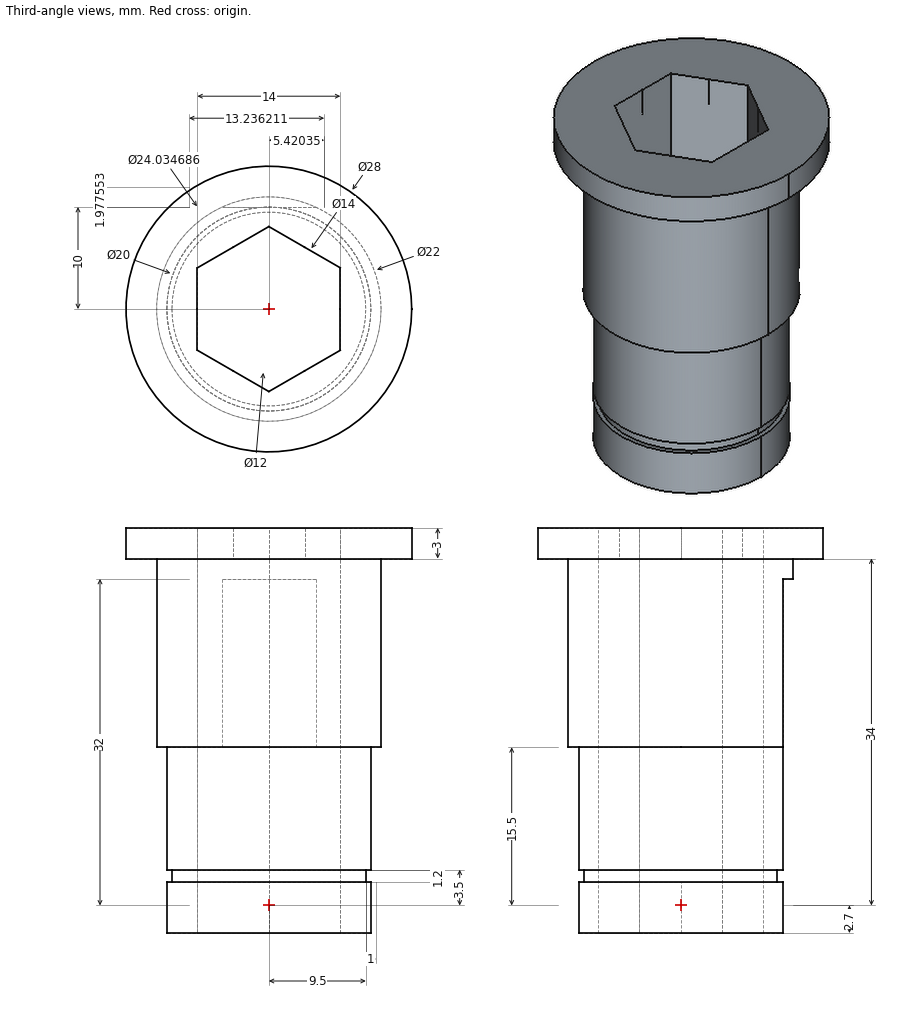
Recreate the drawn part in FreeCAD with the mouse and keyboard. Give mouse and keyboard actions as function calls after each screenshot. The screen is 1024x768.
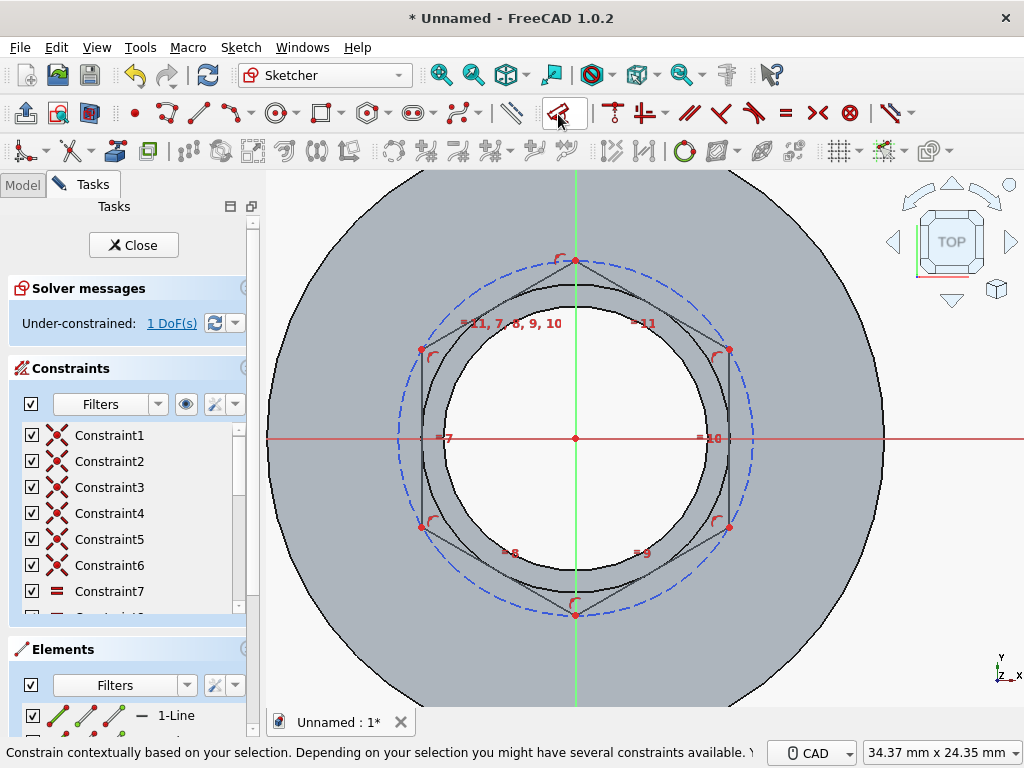
click(422, 350)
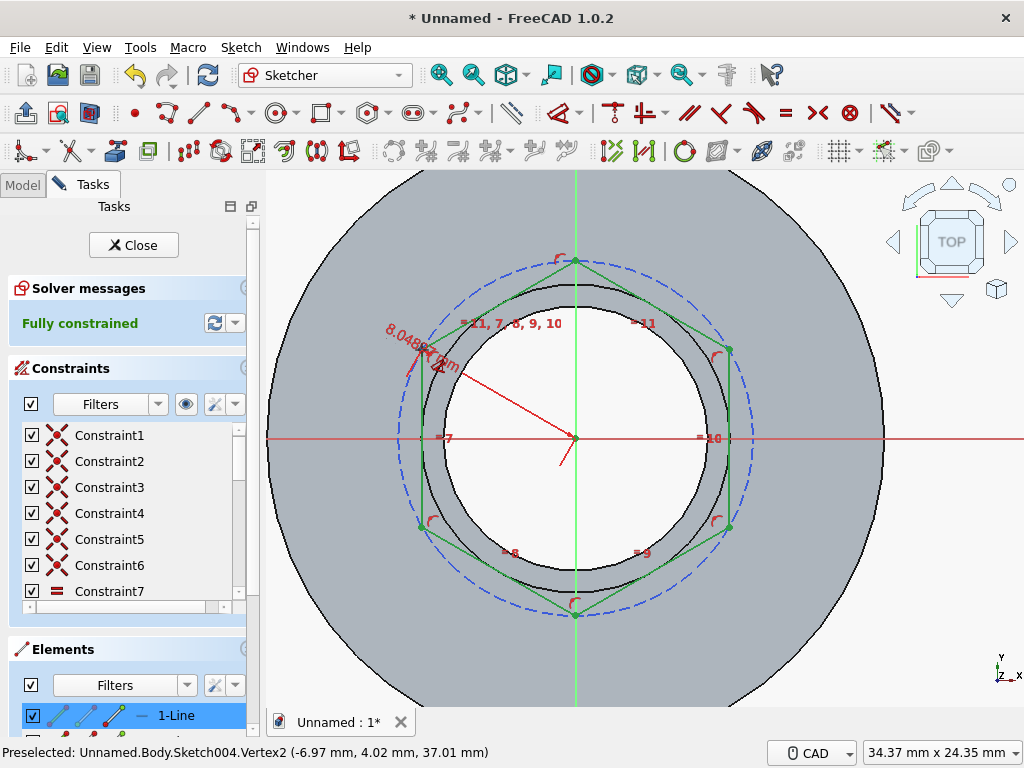
click(729, 527)
click(468, 609)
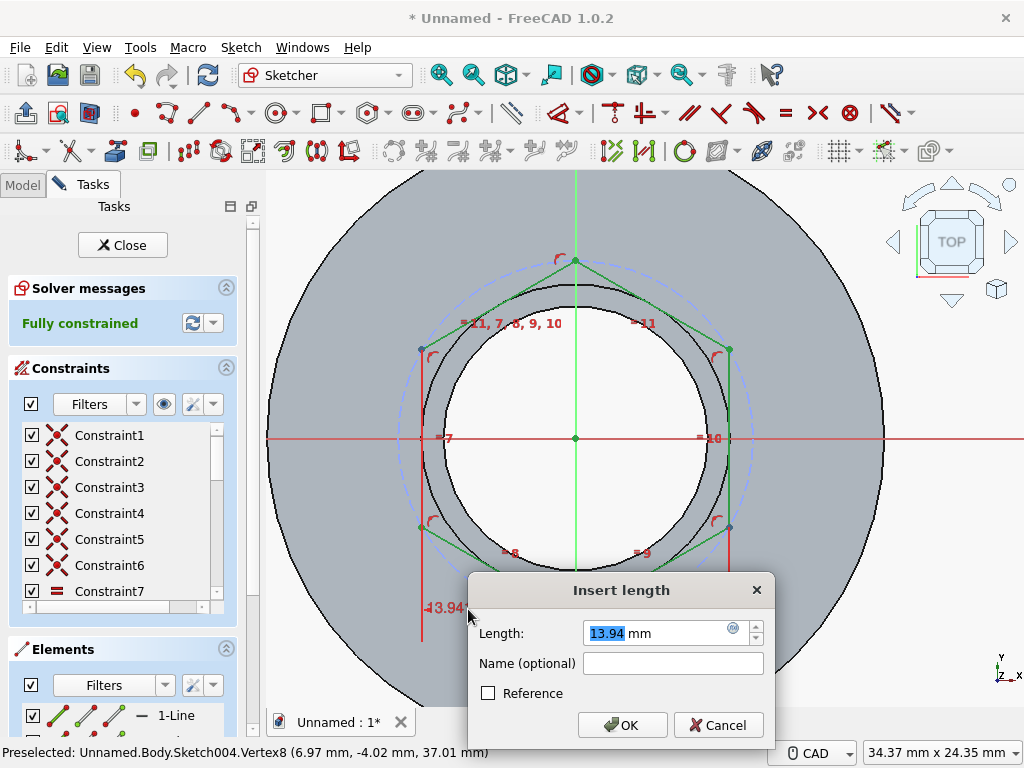
text(14)
key(Return)
key(Escape)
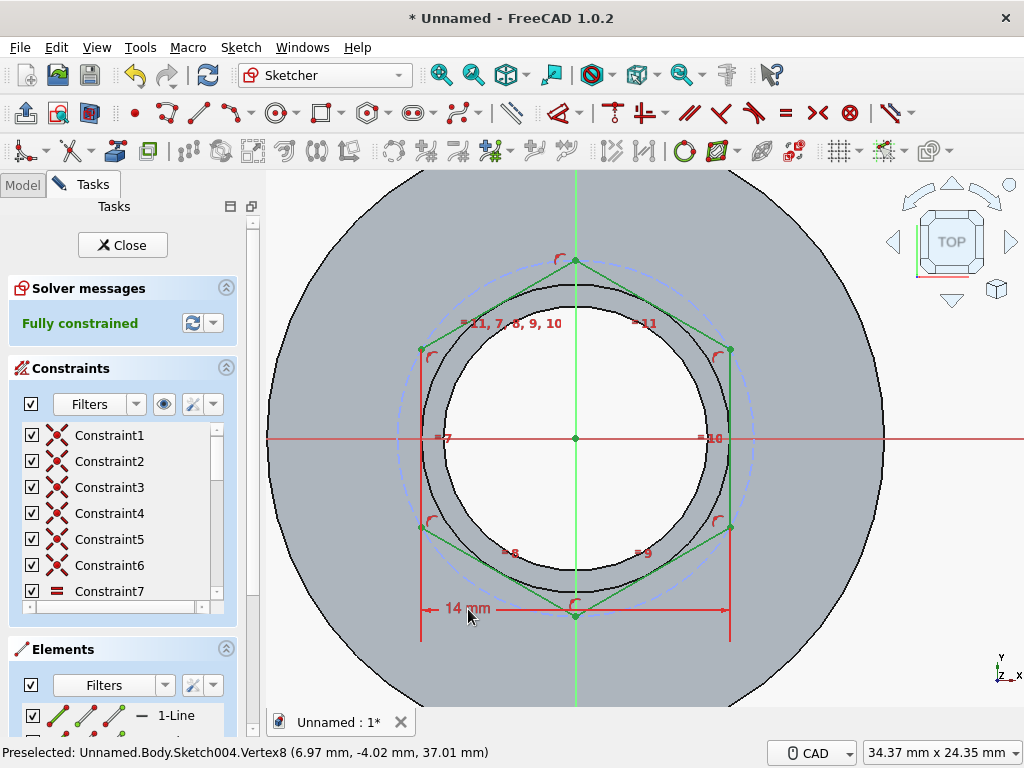
click(123, 245)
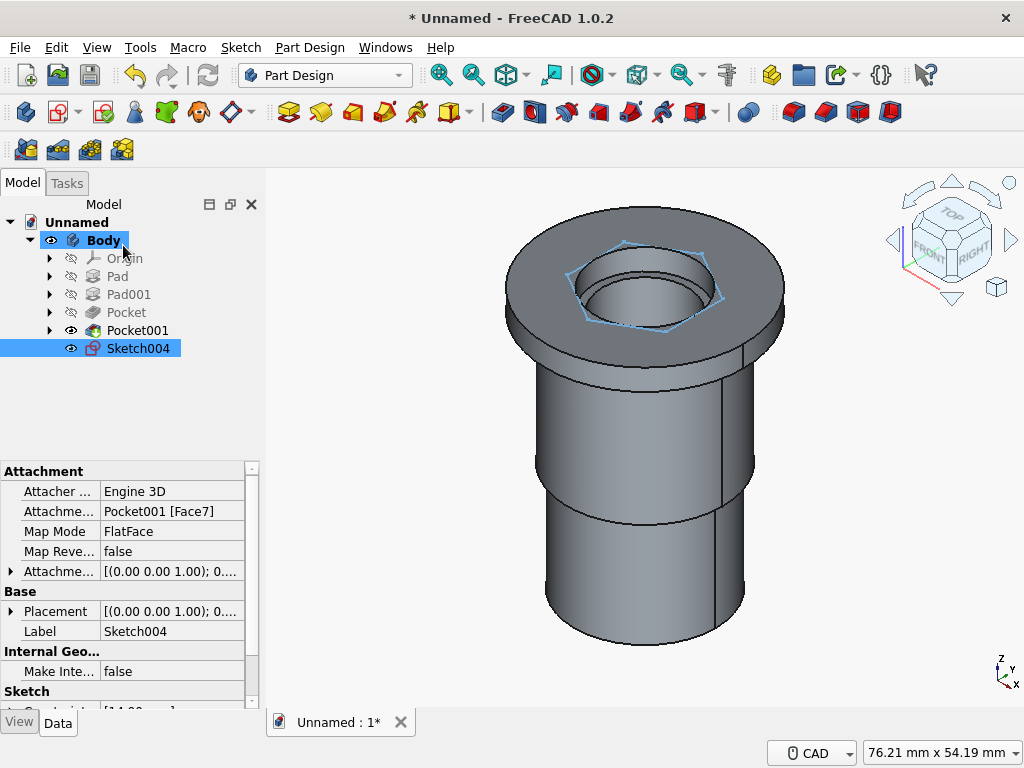
click(504, 112)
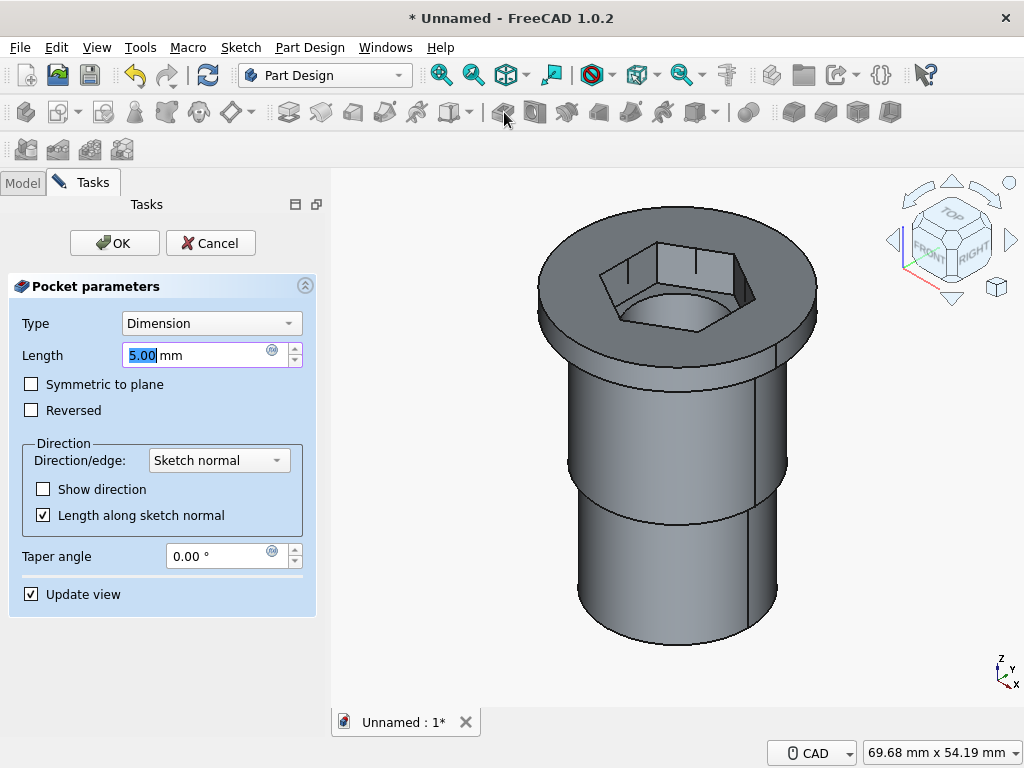
click(212, 324)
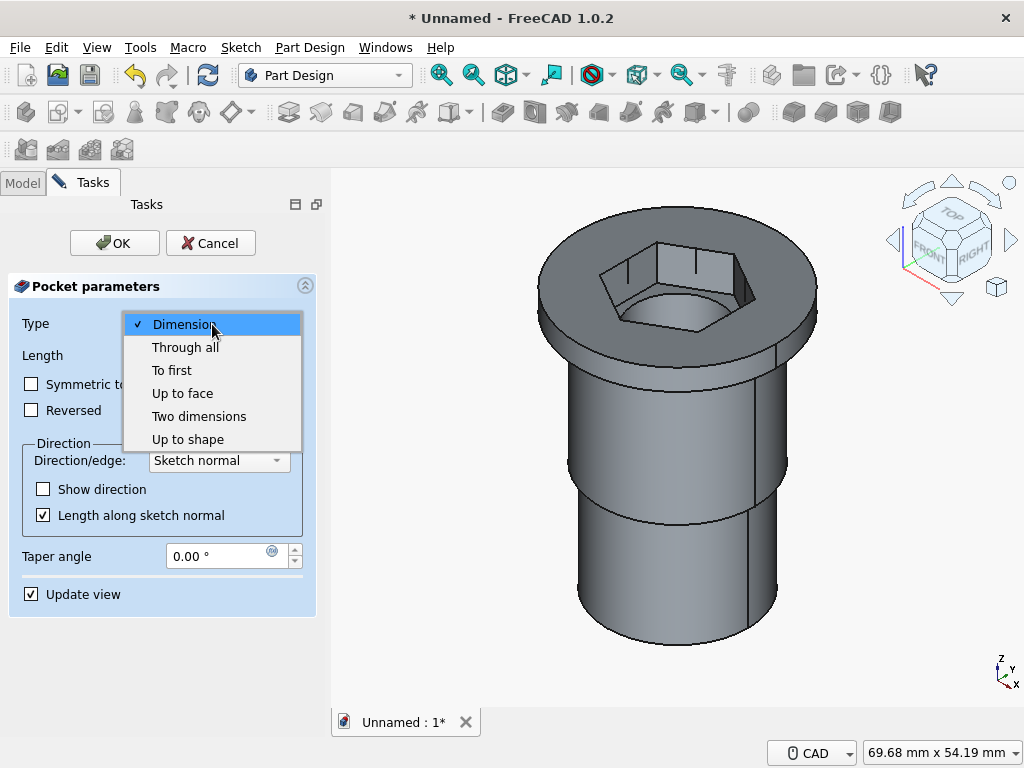
click(212, 348)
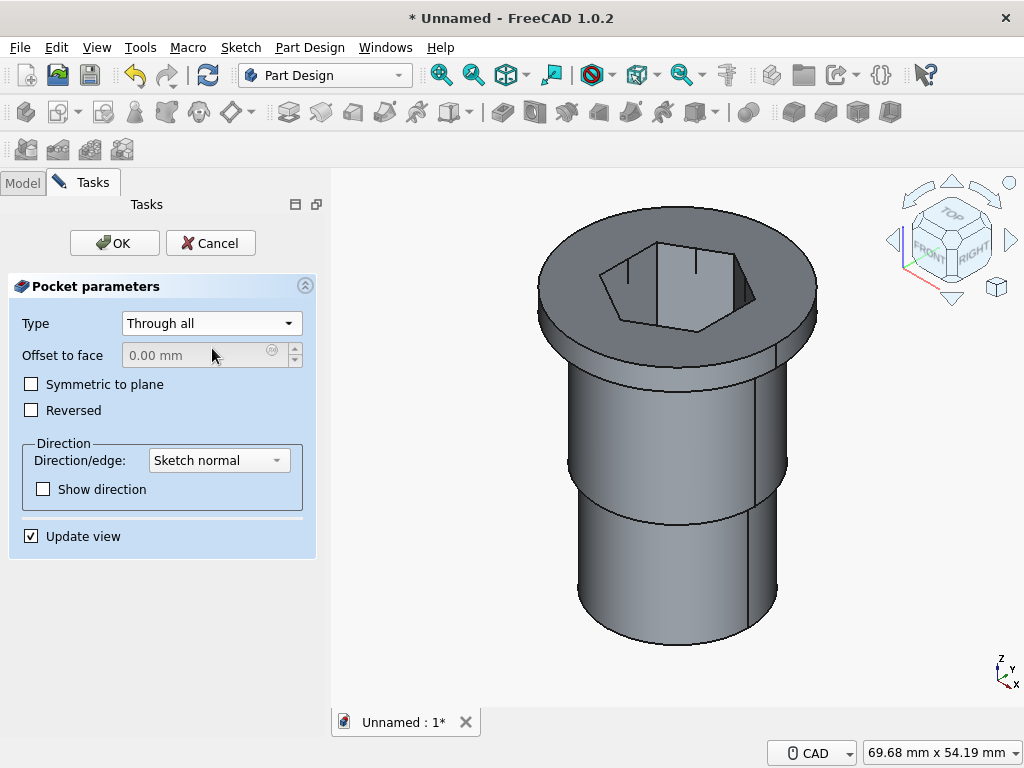
click(115, 243)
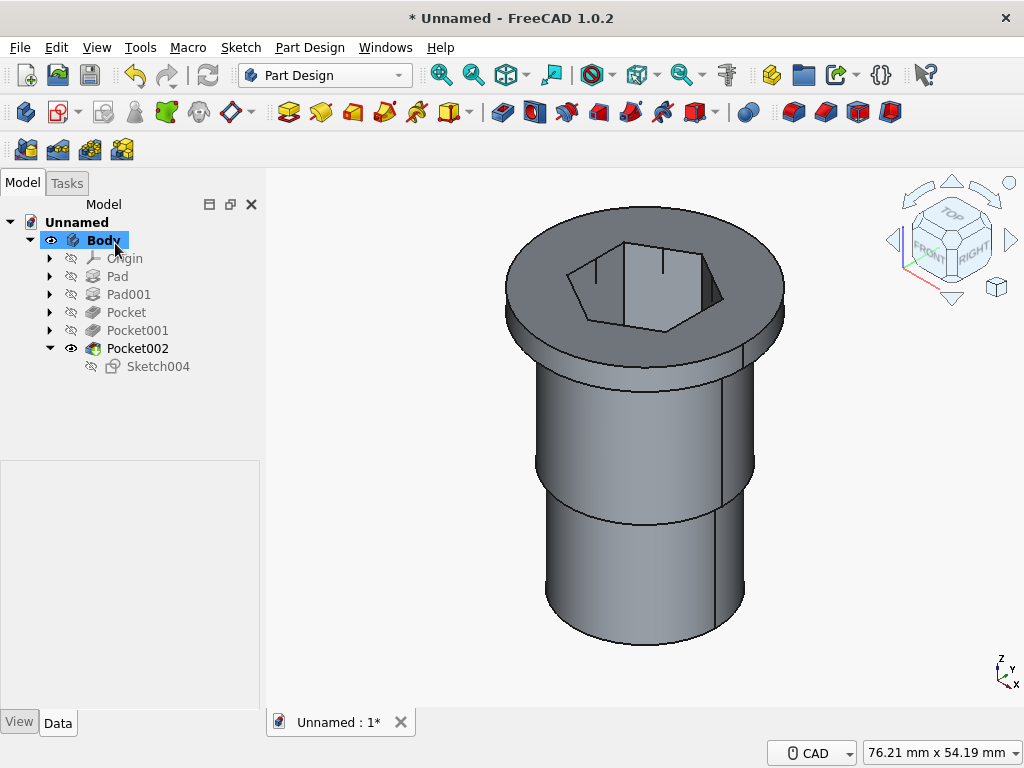
click(58, 112)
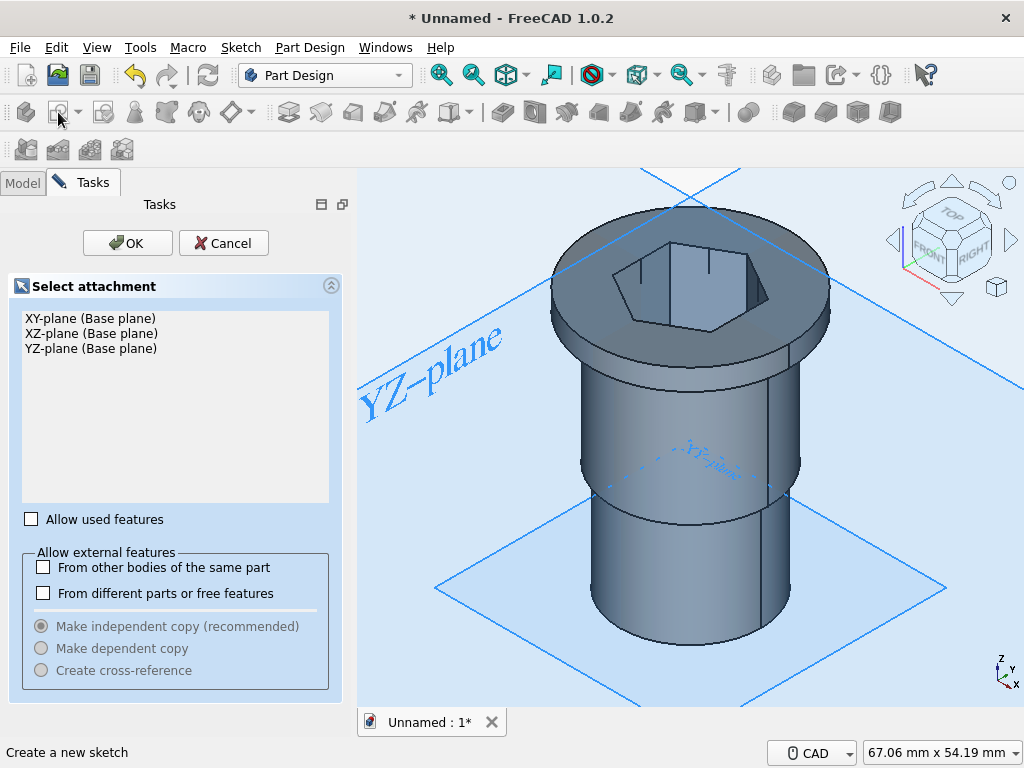
click(82, 334)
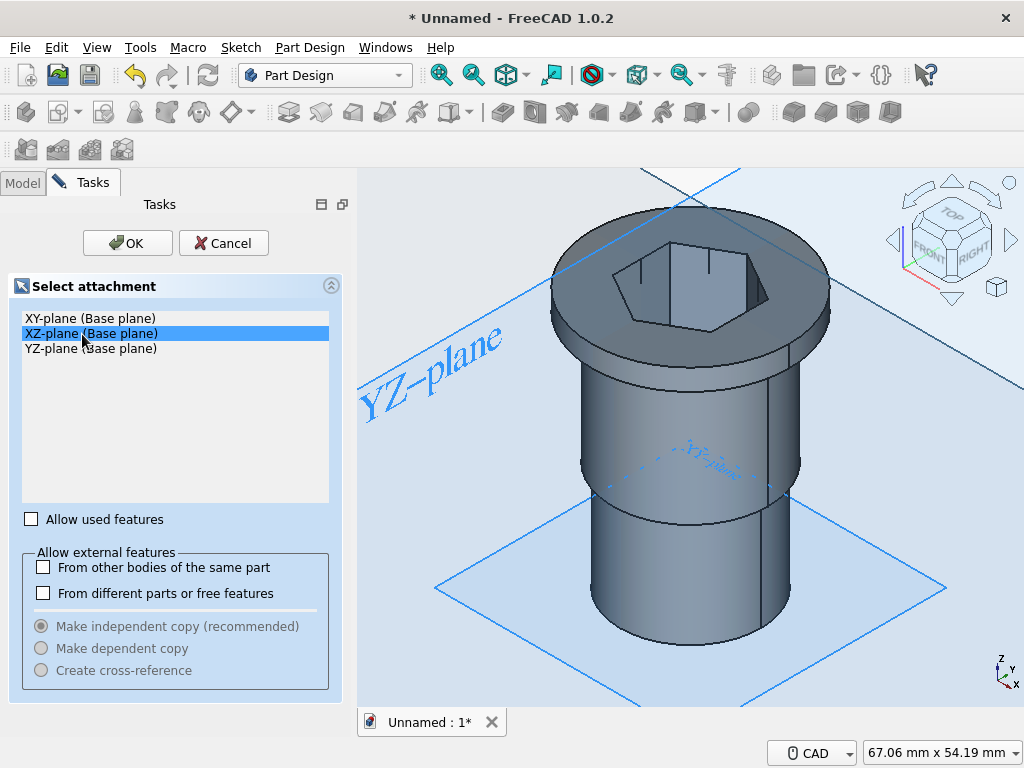
click(128, 243)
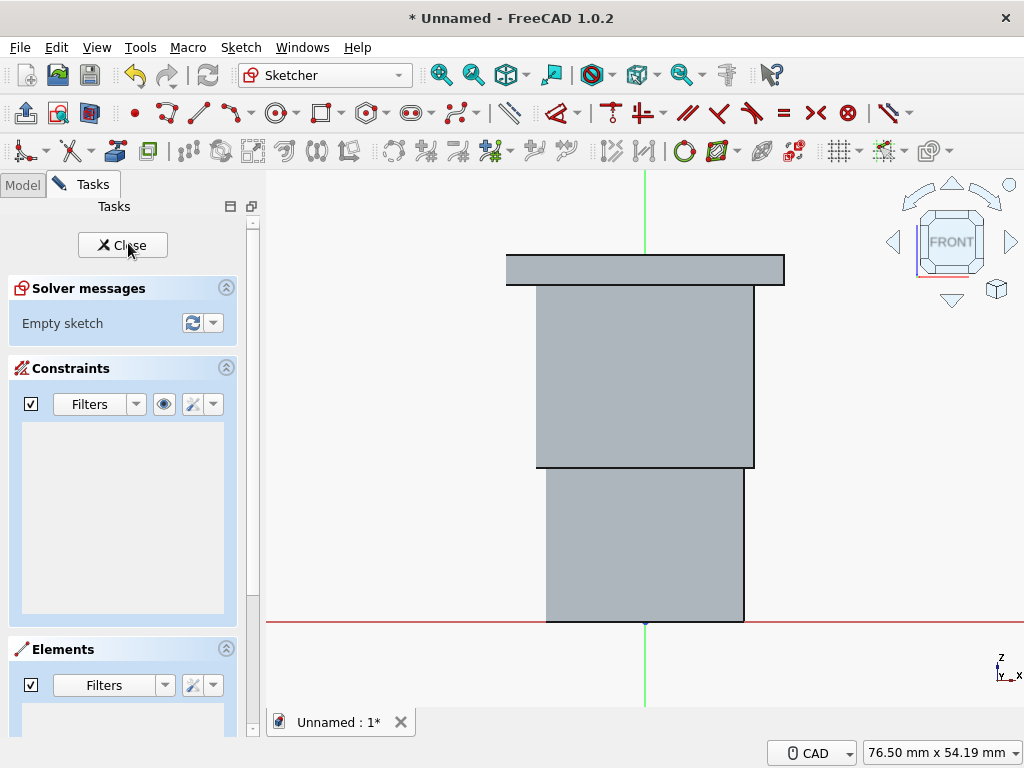
click(90, 114)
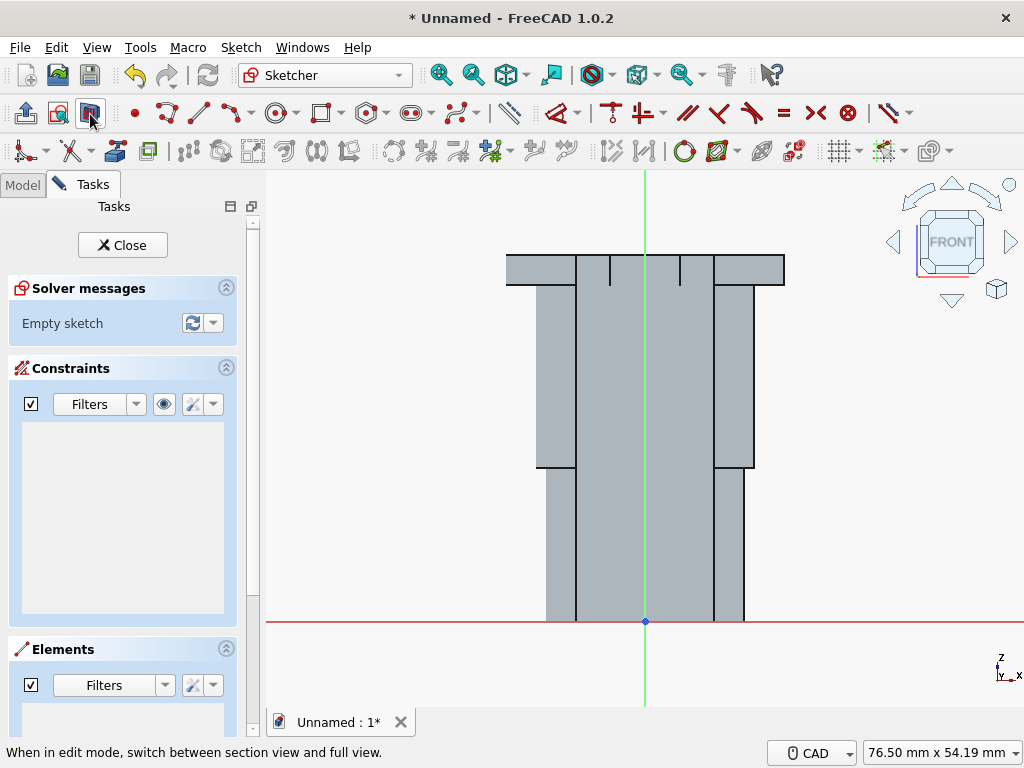
scroll(753, 601, up, 15)